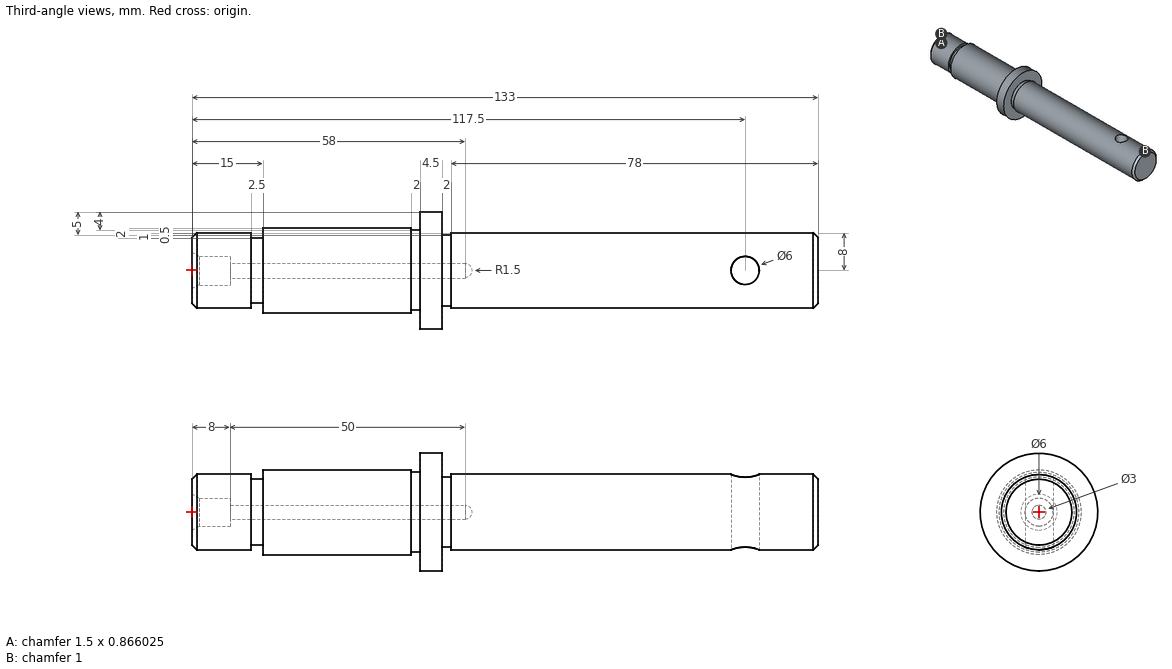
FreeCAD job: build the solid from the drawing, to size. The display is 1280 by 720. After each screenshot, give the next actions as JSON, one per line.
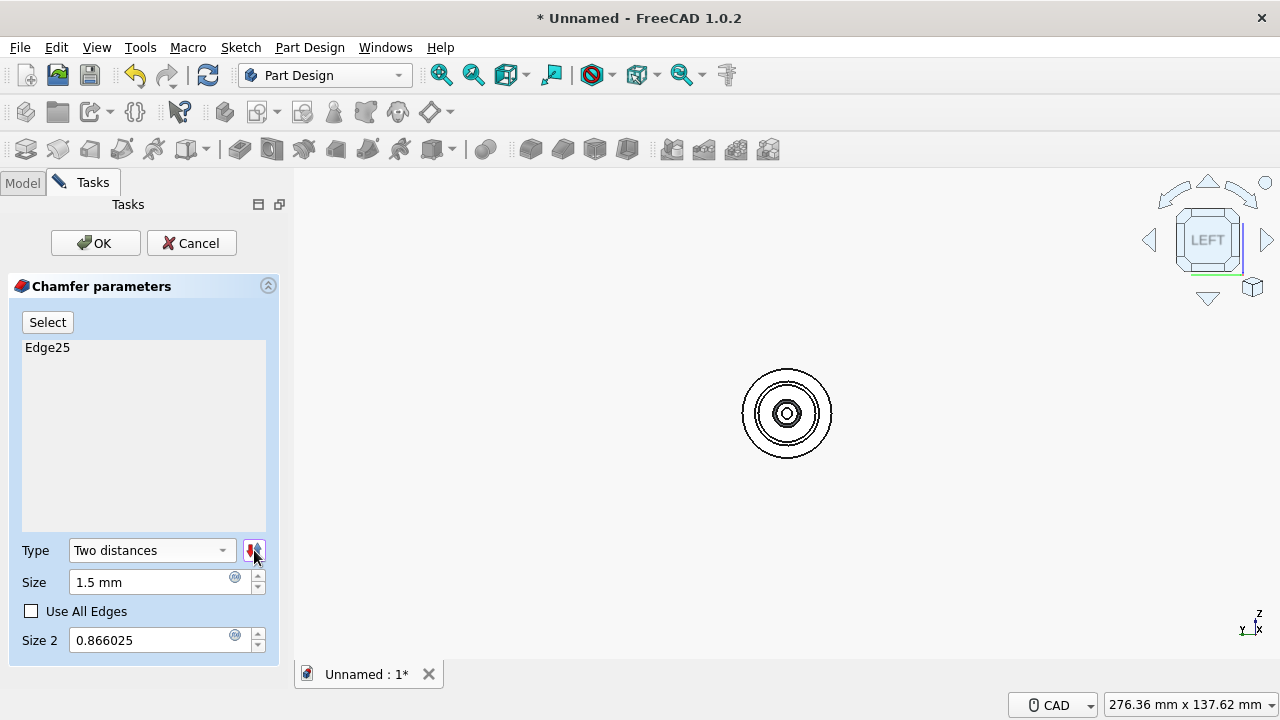
{"action": "left_click", "coordinate": [96, 243]}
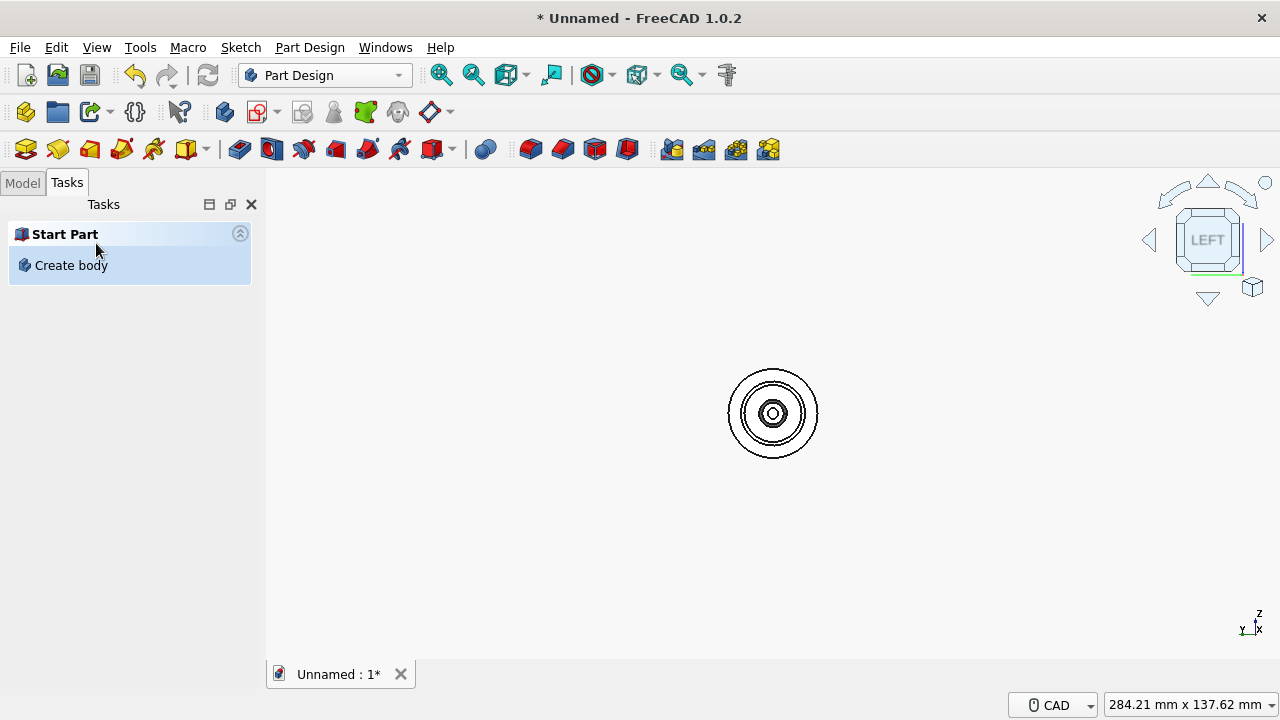
{"action": "left_click", "coordinate": [442, 76]}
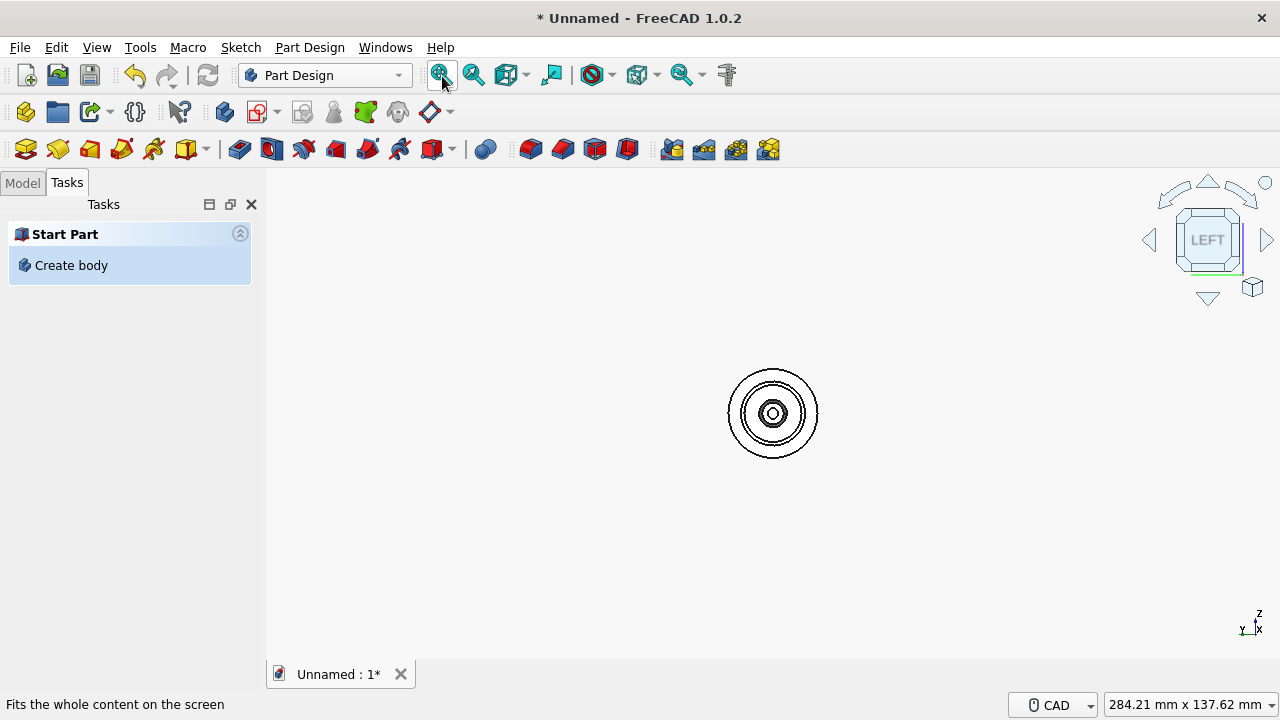
{"action": "left_click", "coordinate": [796, 396]}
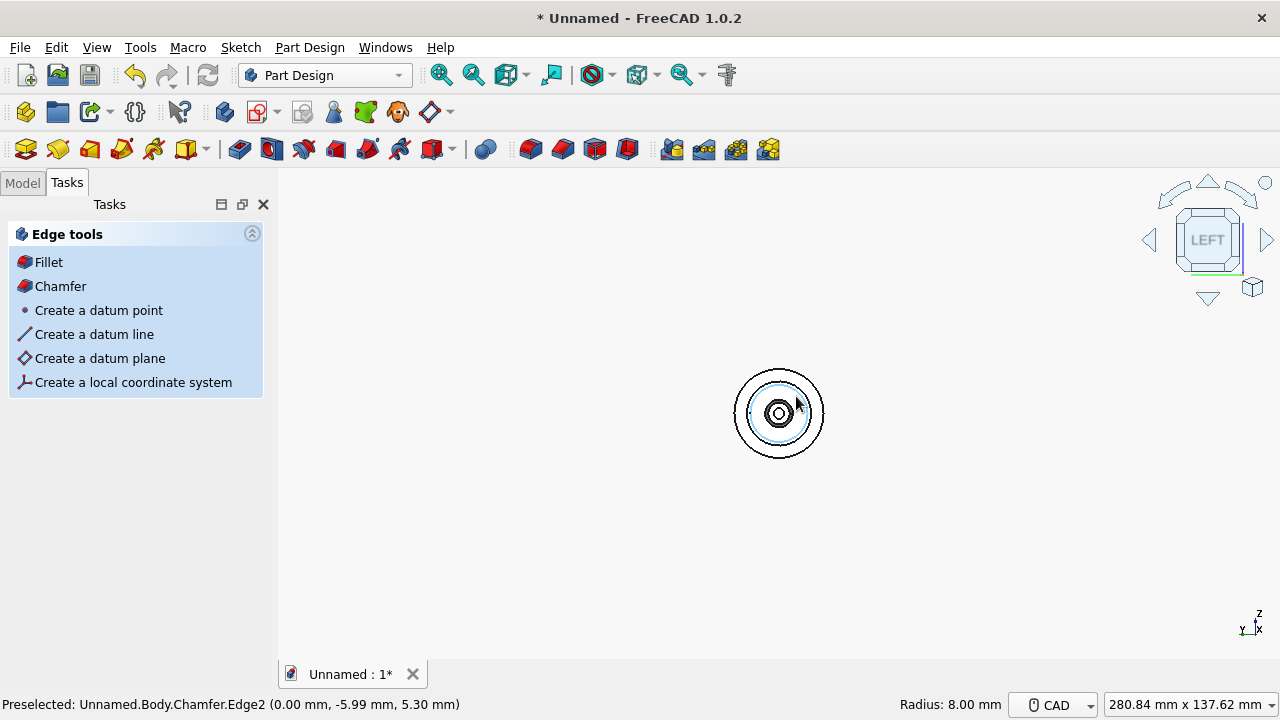
{"action": "key", "text": "0"}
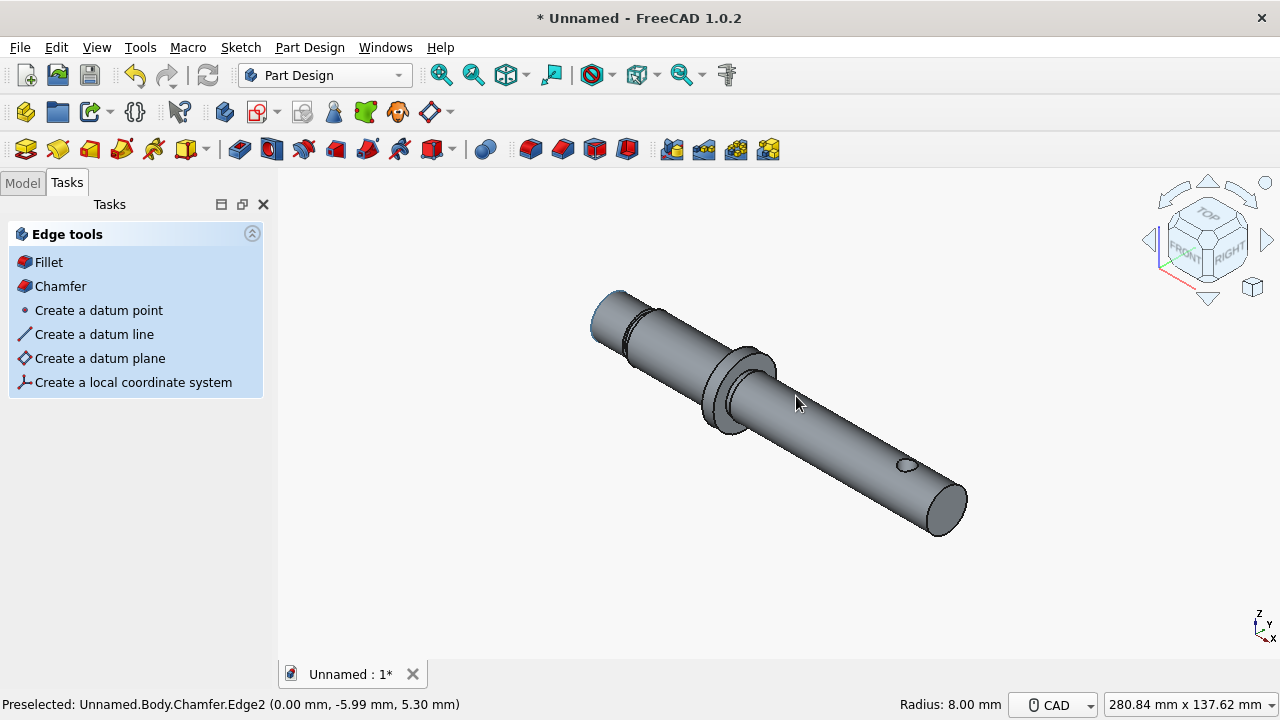
{"action": "left_click", "coordinate": [927, 521], "text": "ctrl"}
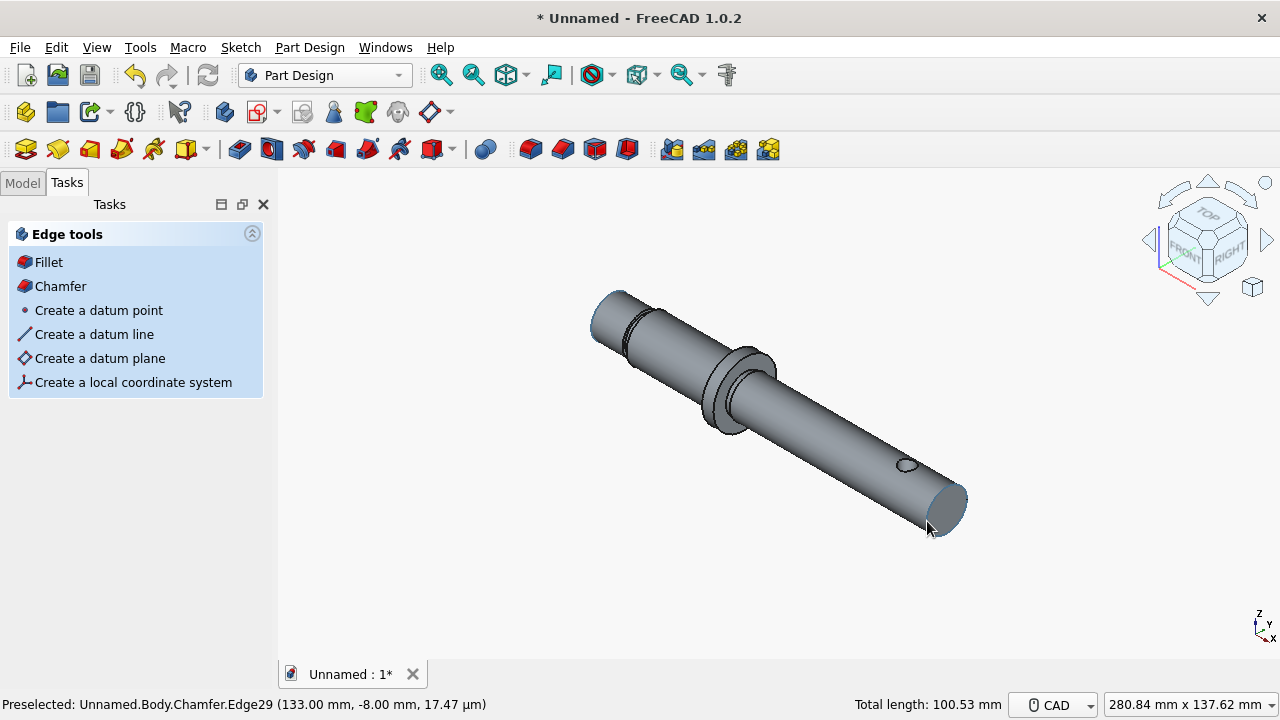
{"action": "left_click", "coordinate": [564, 150]}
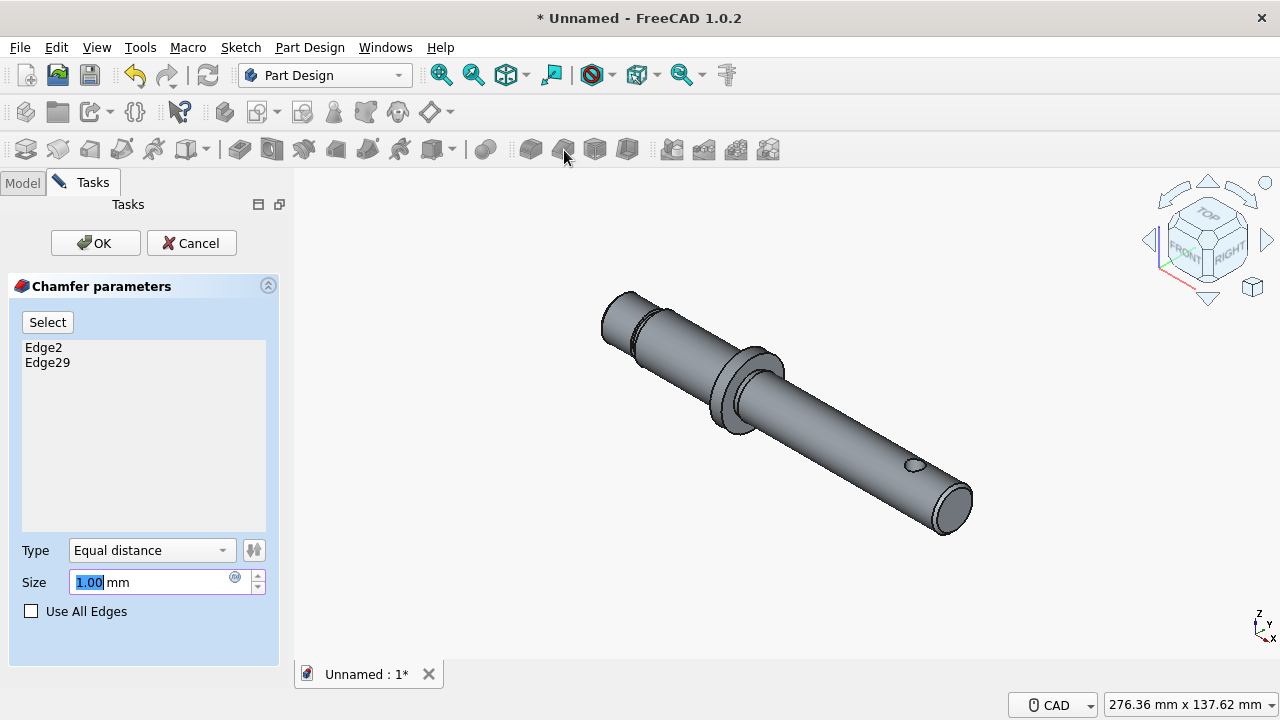
{"action": "type", "text": "1"}
{"action": "key", "text": "Tab"}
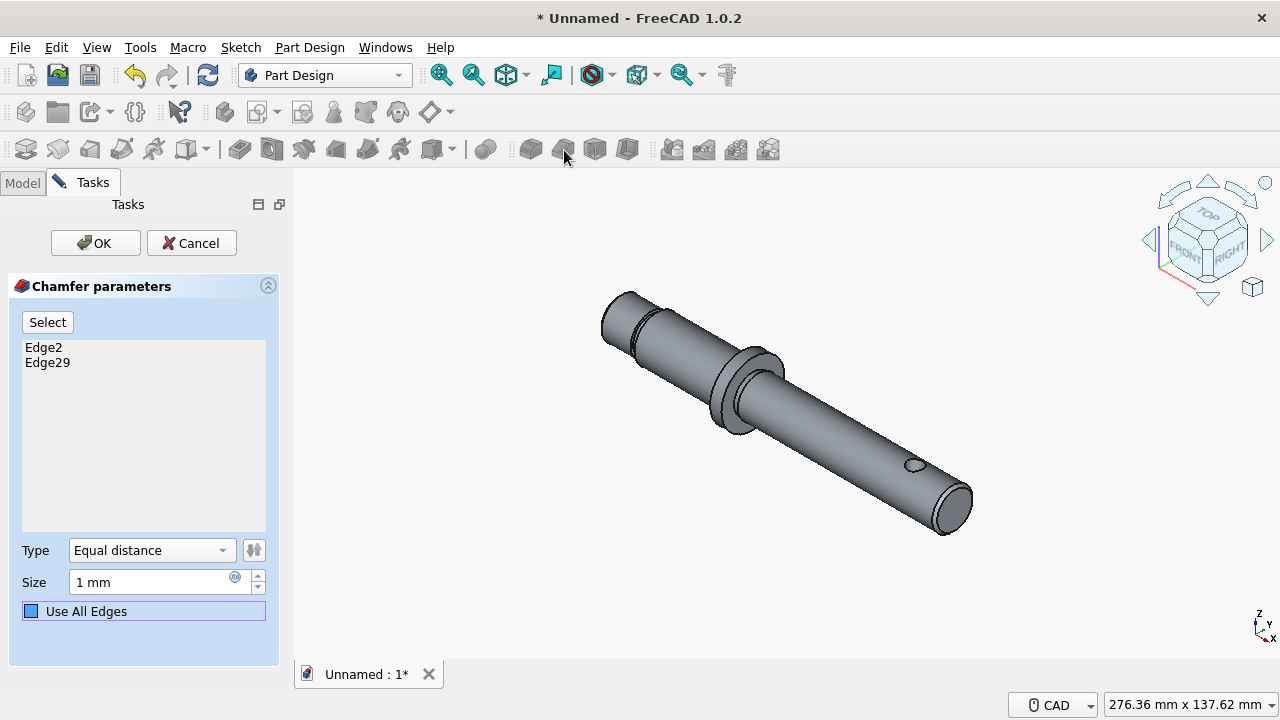
{"action": "left_click", "coordinate": [96, 243]}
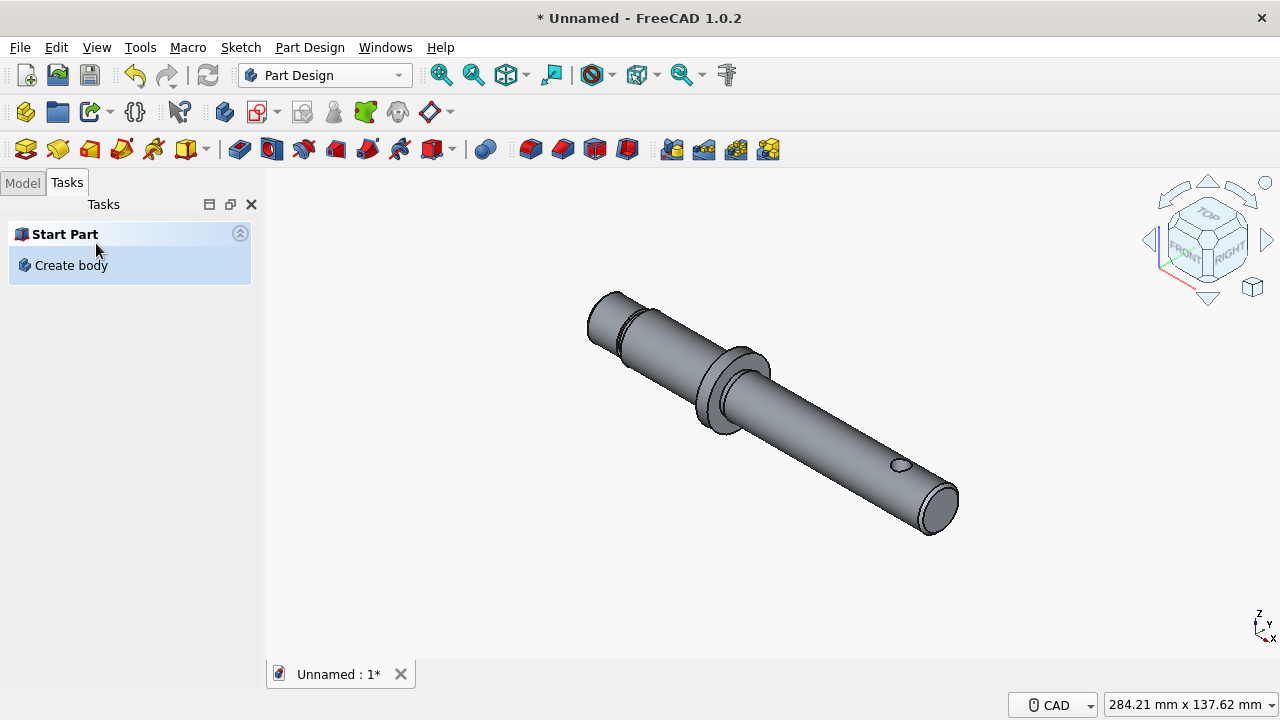
{"action": "left_click", "coordinate": [258, 112]}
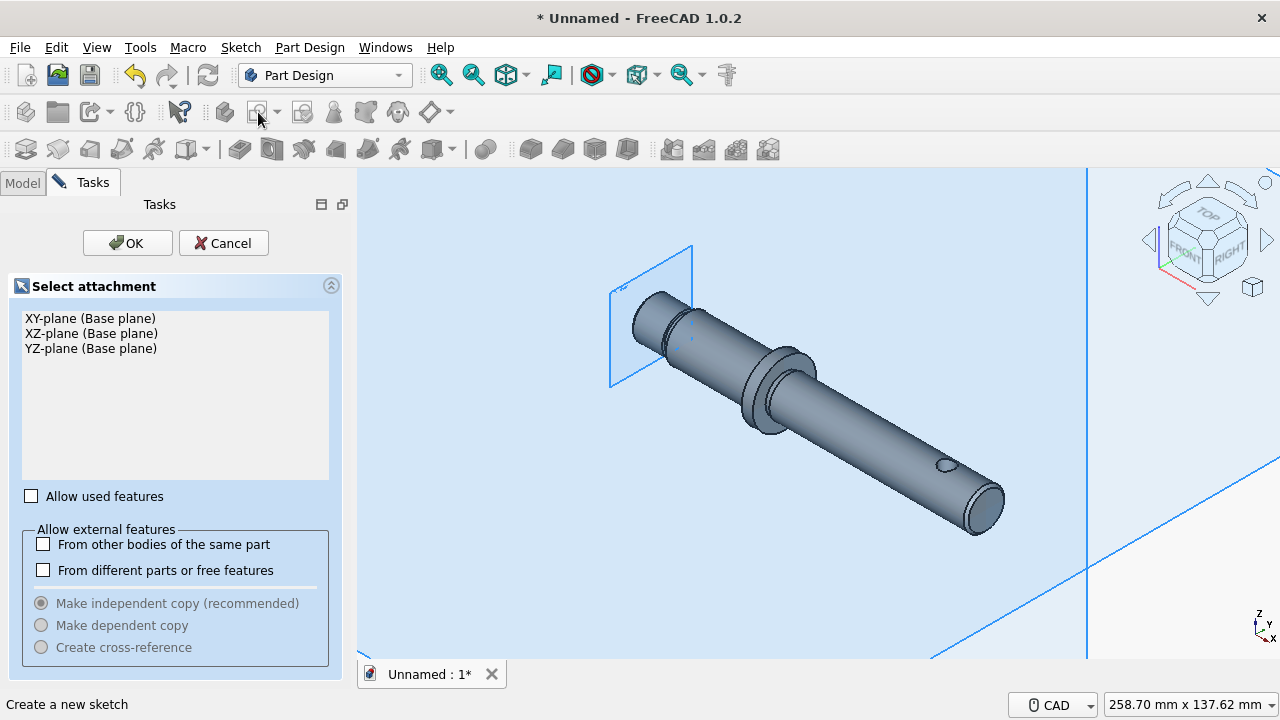
{"action": "left_click", "coordinate": [82, 318]}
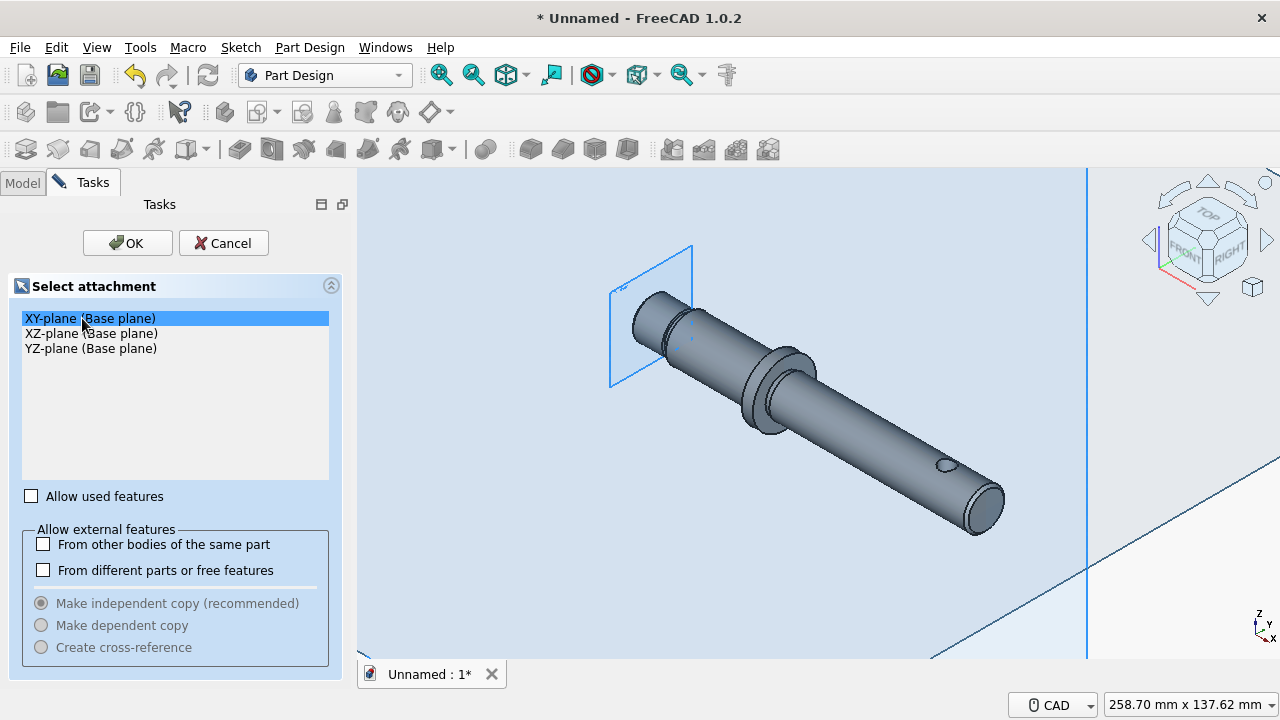
{"action": "left_click", "coordinate": [128, 243]}